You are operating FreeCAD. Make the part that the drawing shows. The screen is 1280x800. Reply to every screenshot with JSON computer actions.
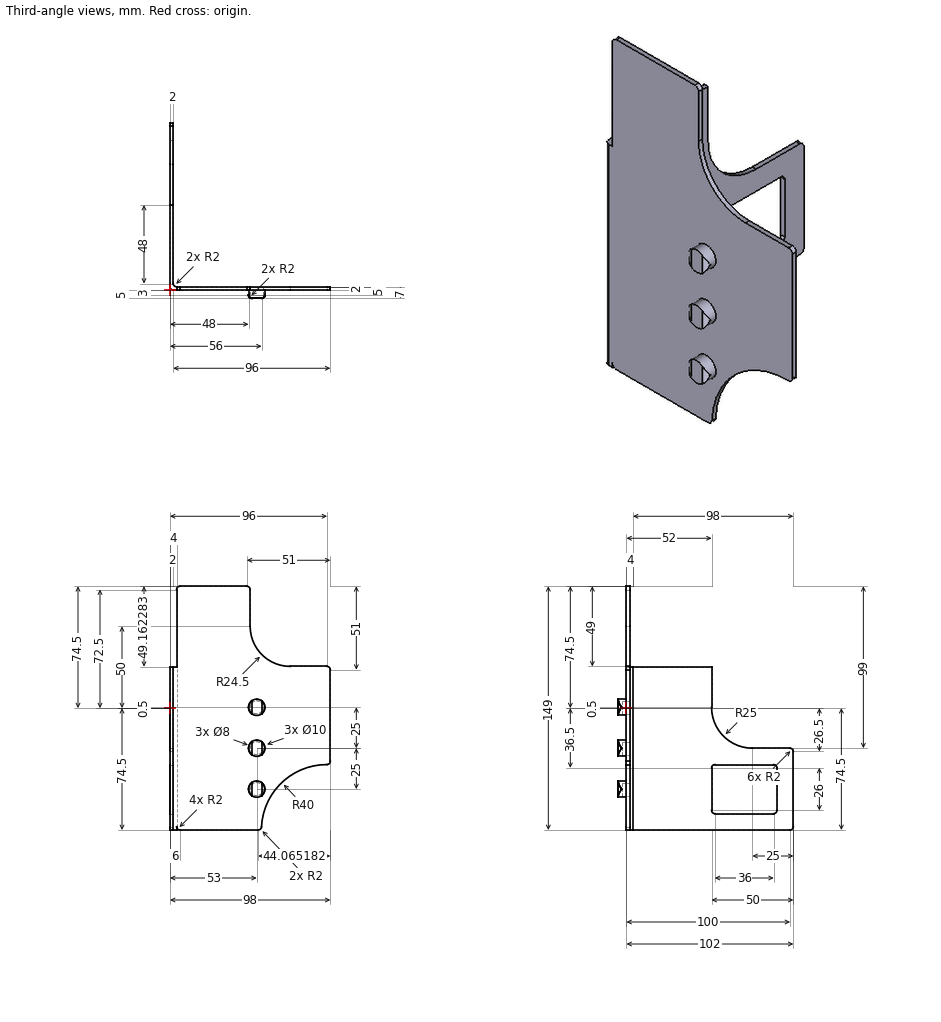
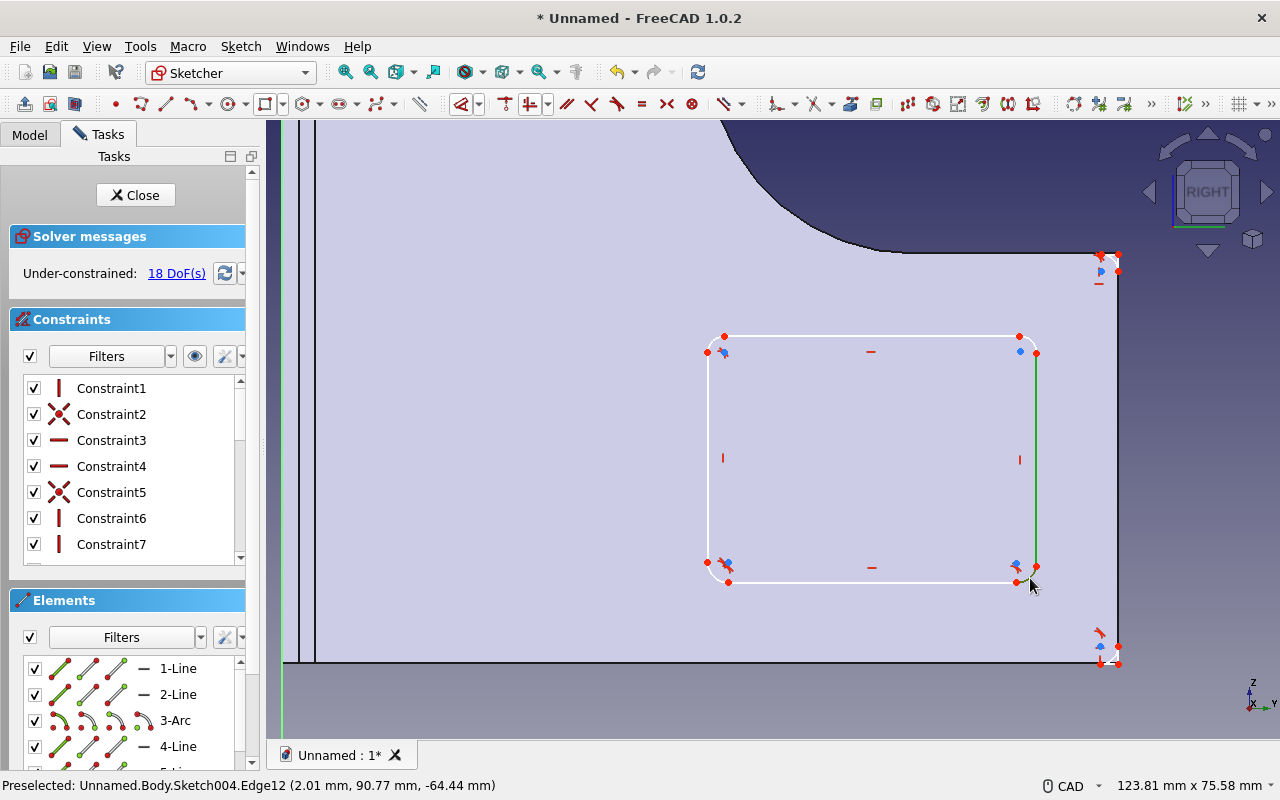
{"action": "key", "text": "t"}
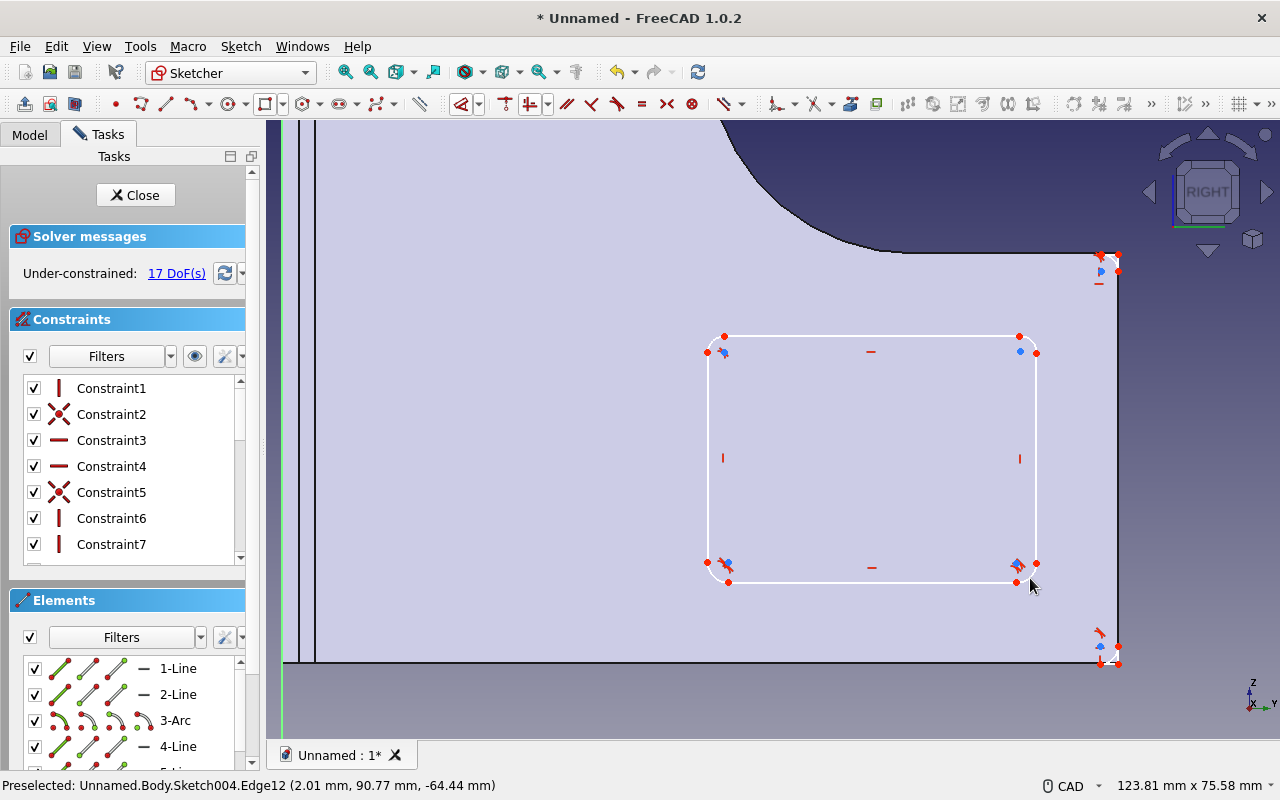
{"action": "left_click", "coordinate": [1036, 500]}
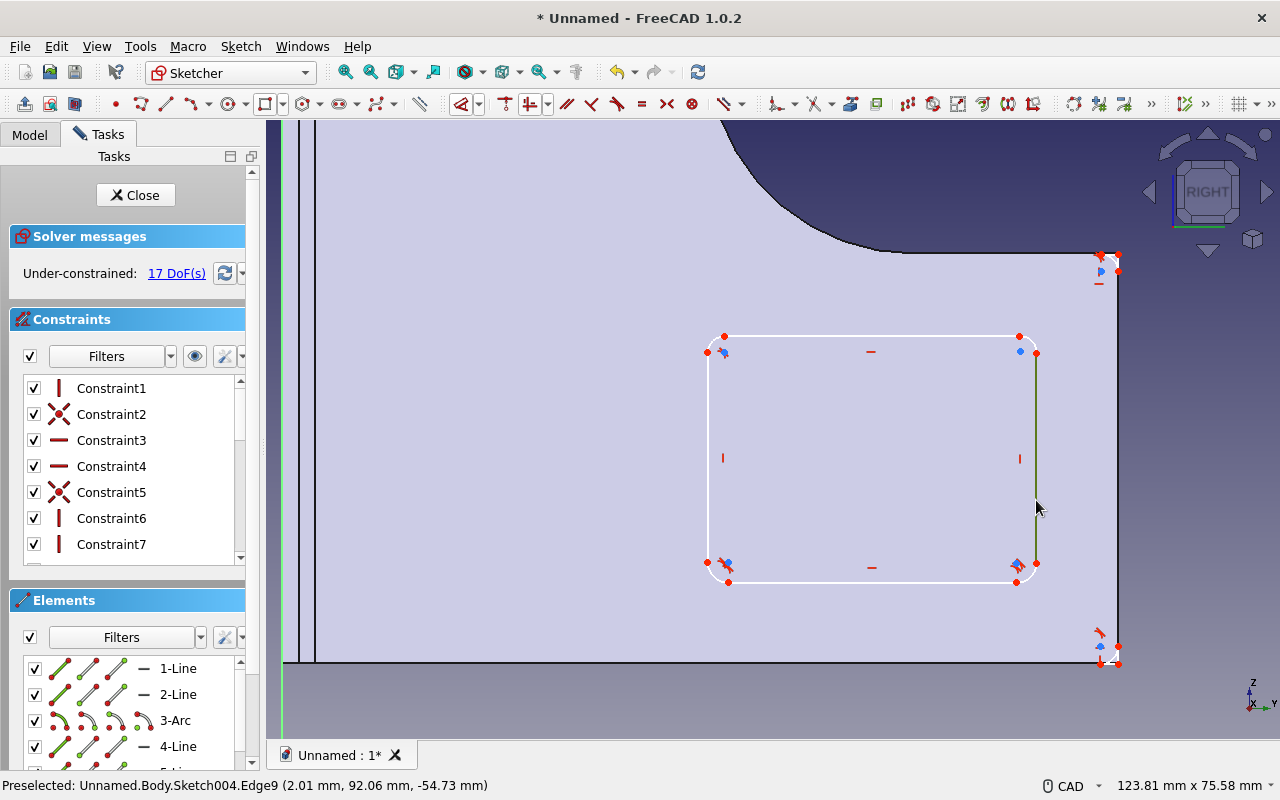
{"action": "left_click", "coordinate": [1032, 341]}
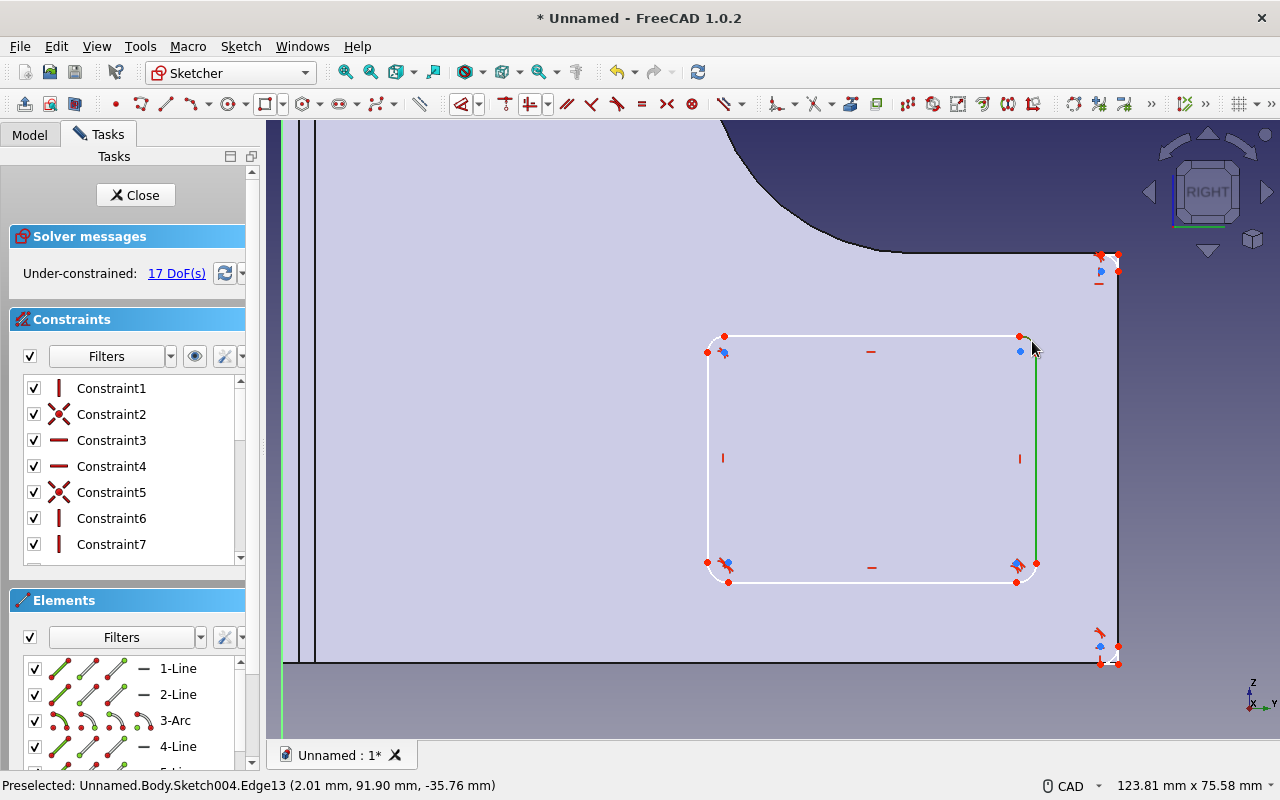
{"action": "key", "text": "t"}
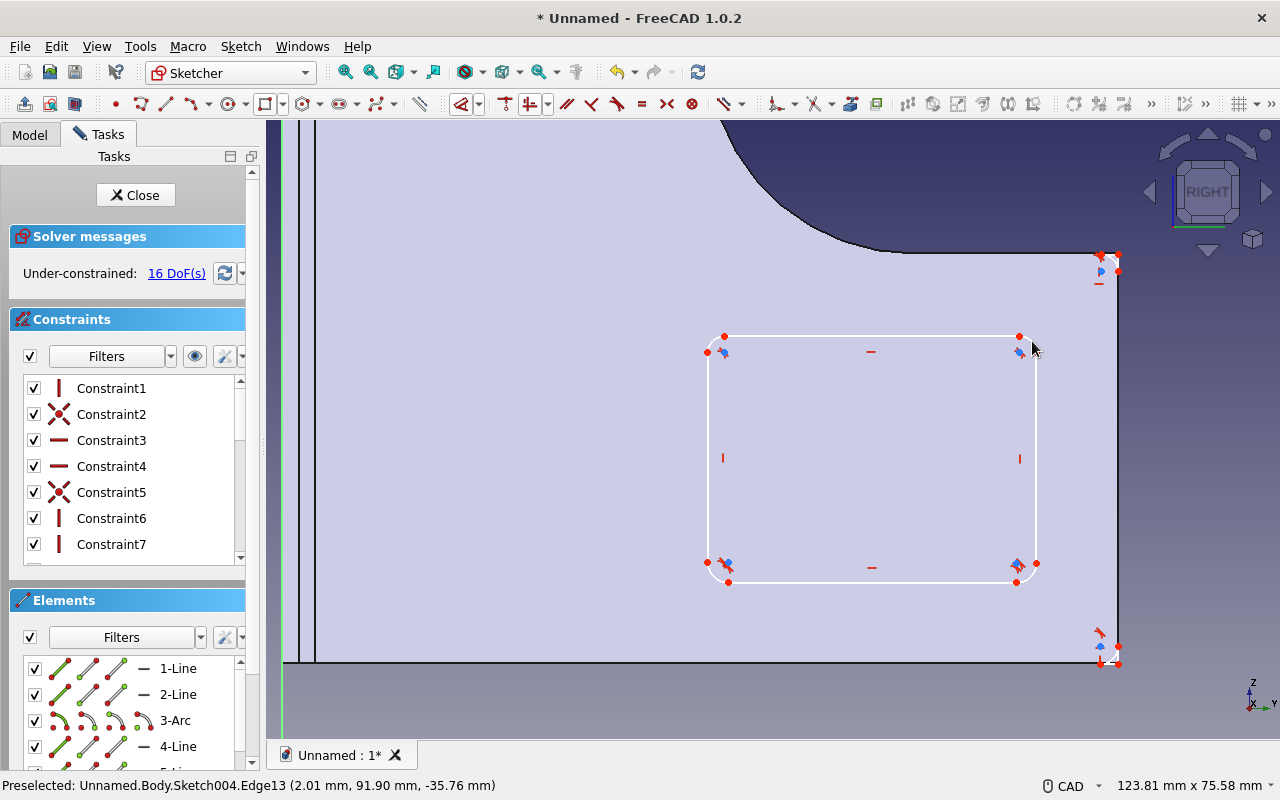
{"action": "left_click", "coordinate": [931, 336]}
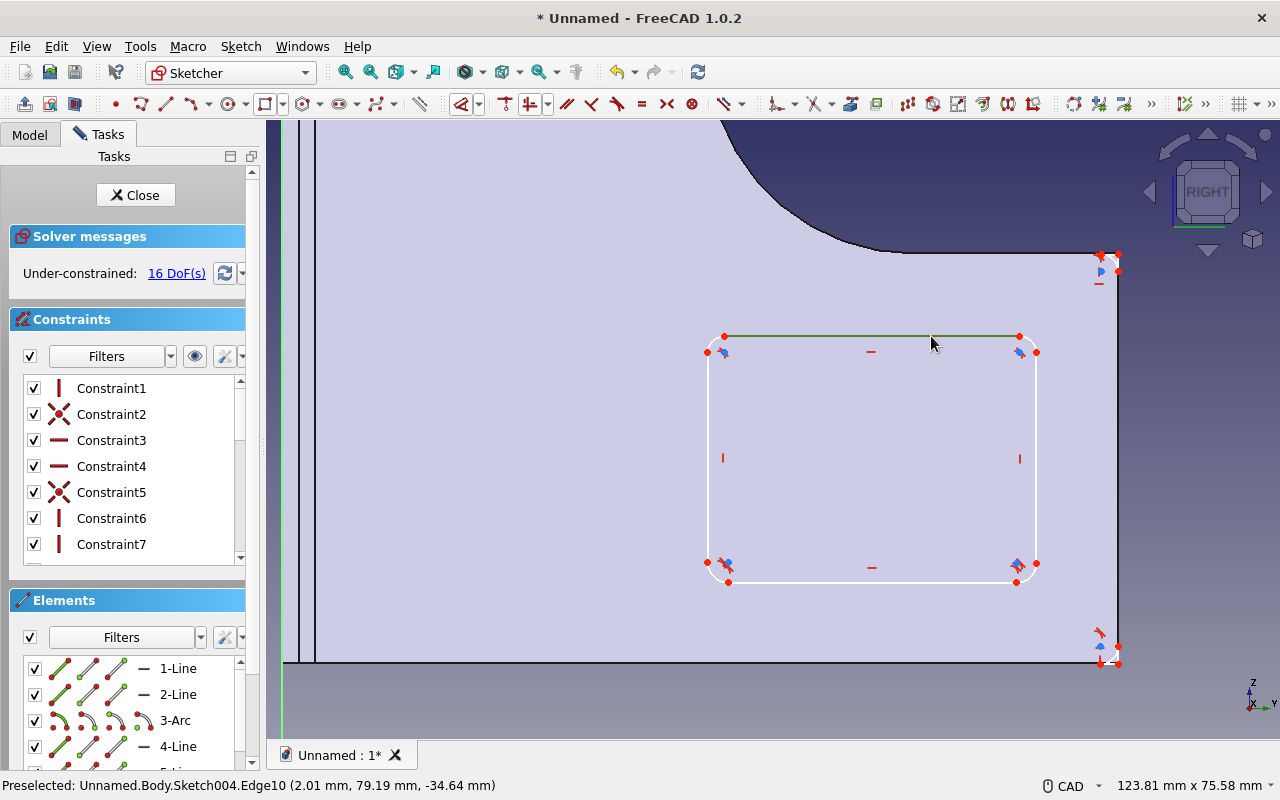
{"action": "left_click", "coordinate": [1031, 341]}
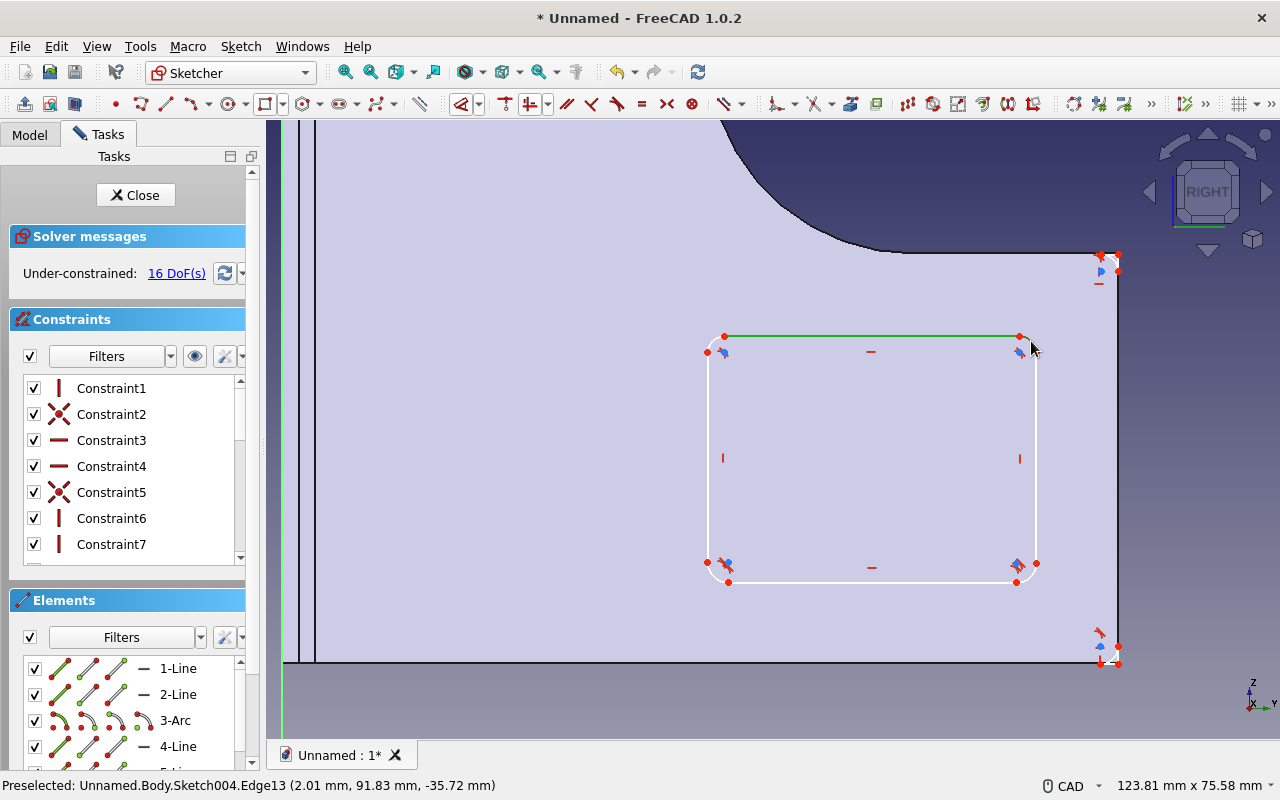
{"action": "left_click", "coordinate": [617, 104]}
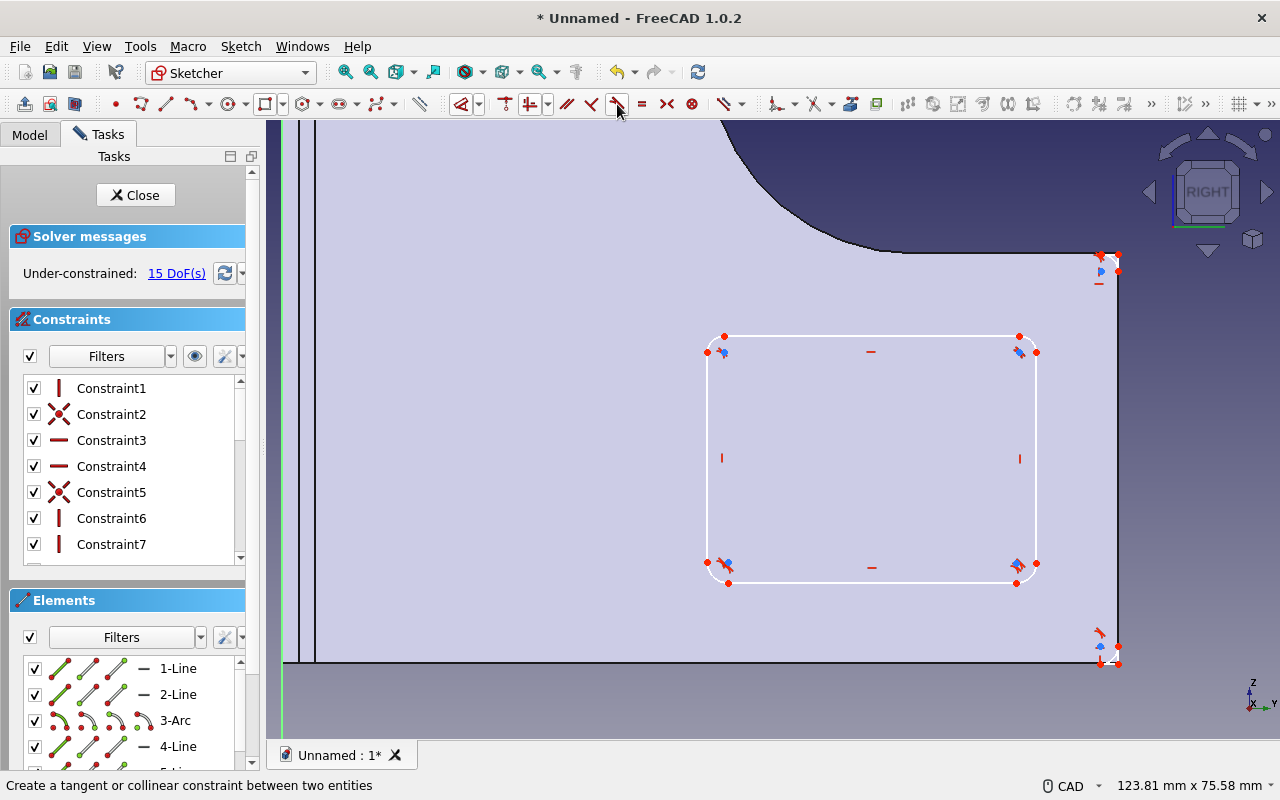
{"action": "left_click", "coordinate": [931, 336]}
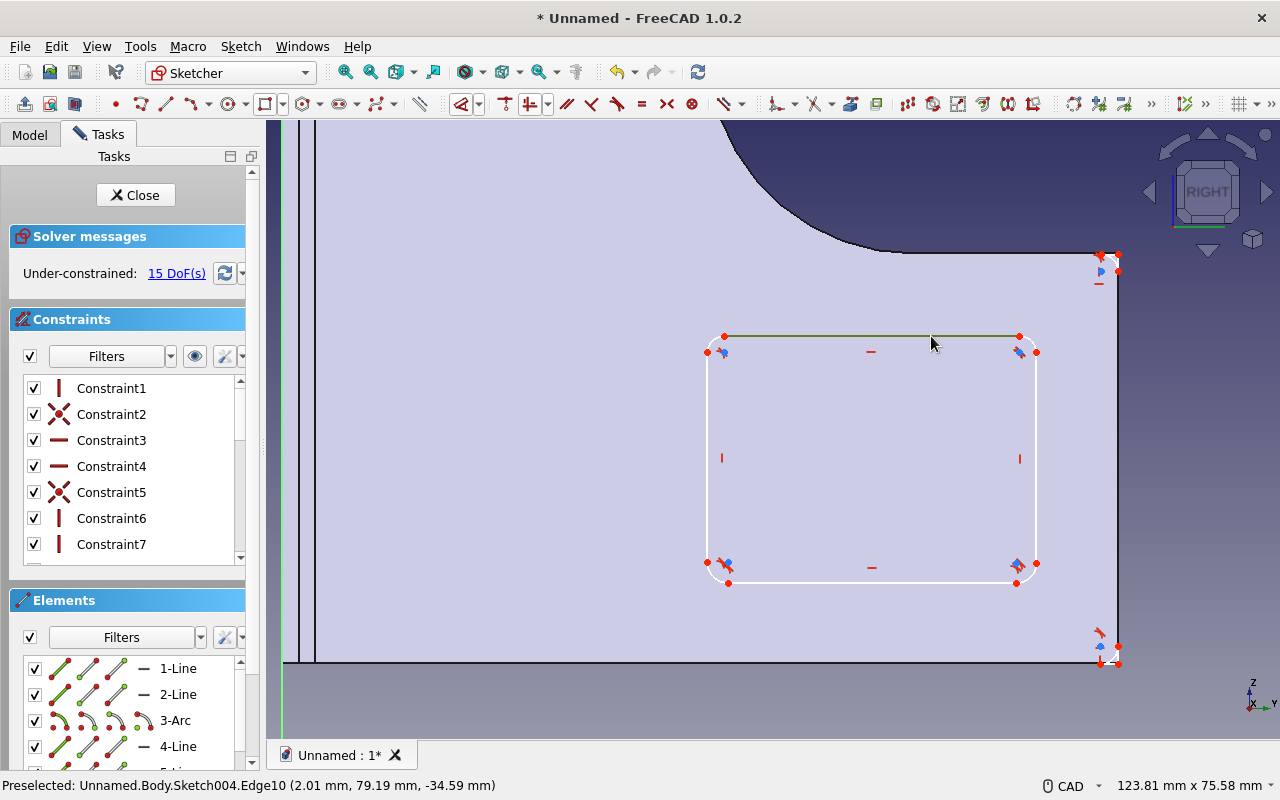
{"action": "left_click", "coordinate": [712, 341]}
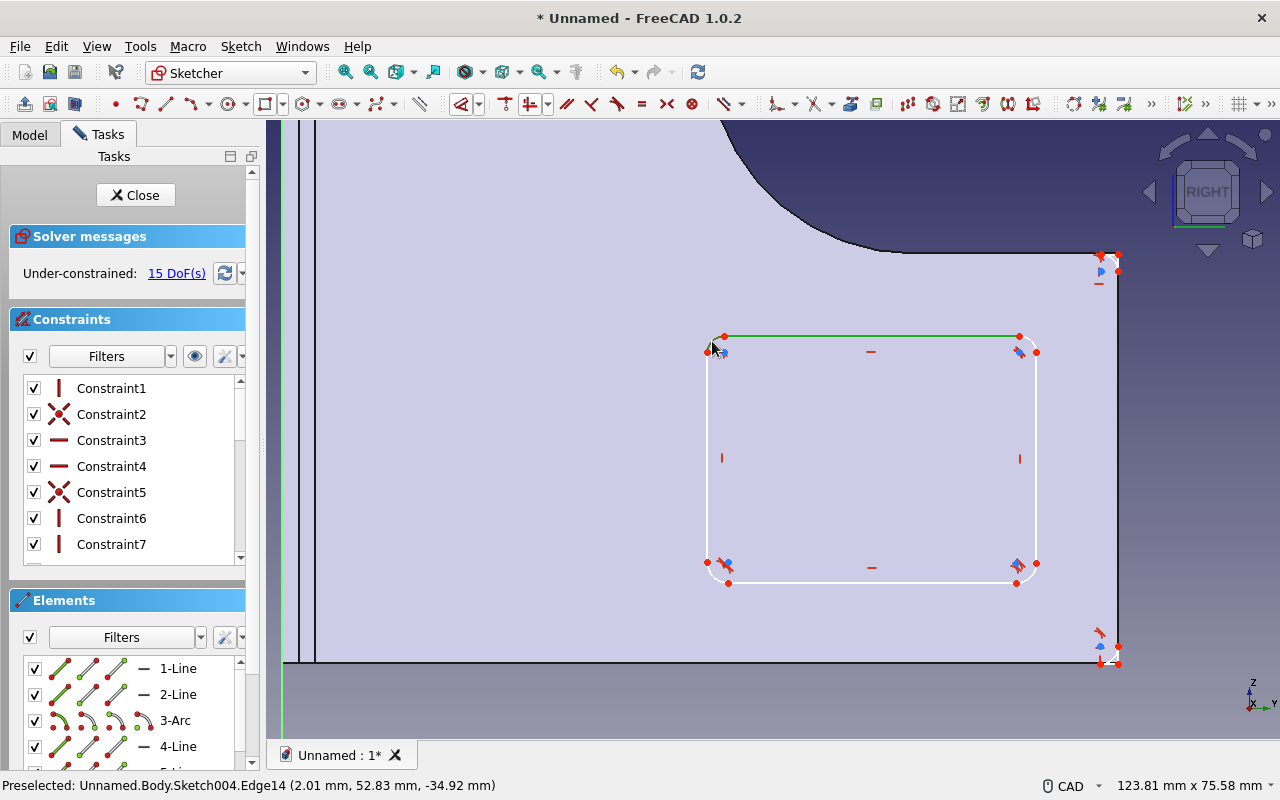
{"action": "key", "text": "t"}